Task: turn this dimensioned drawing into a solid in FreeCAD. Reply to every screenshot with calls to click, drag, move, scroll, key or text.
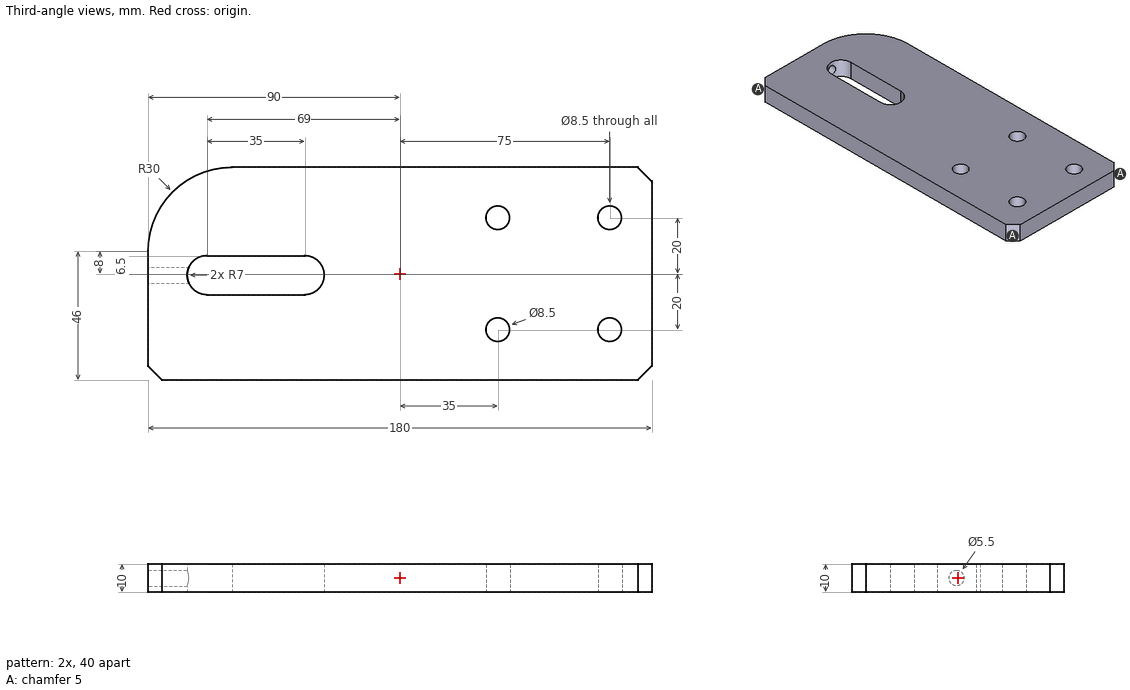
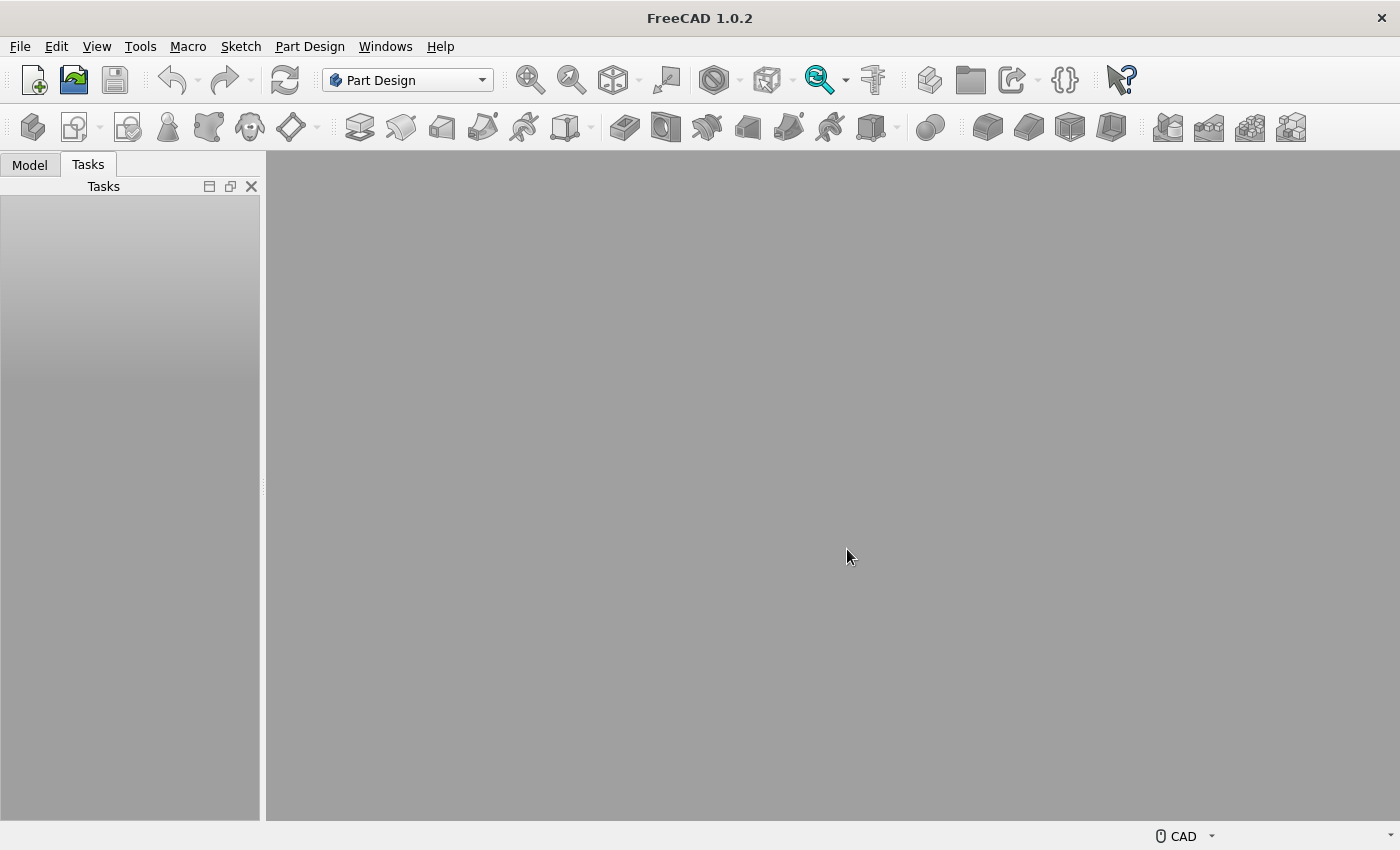
click(33, 80)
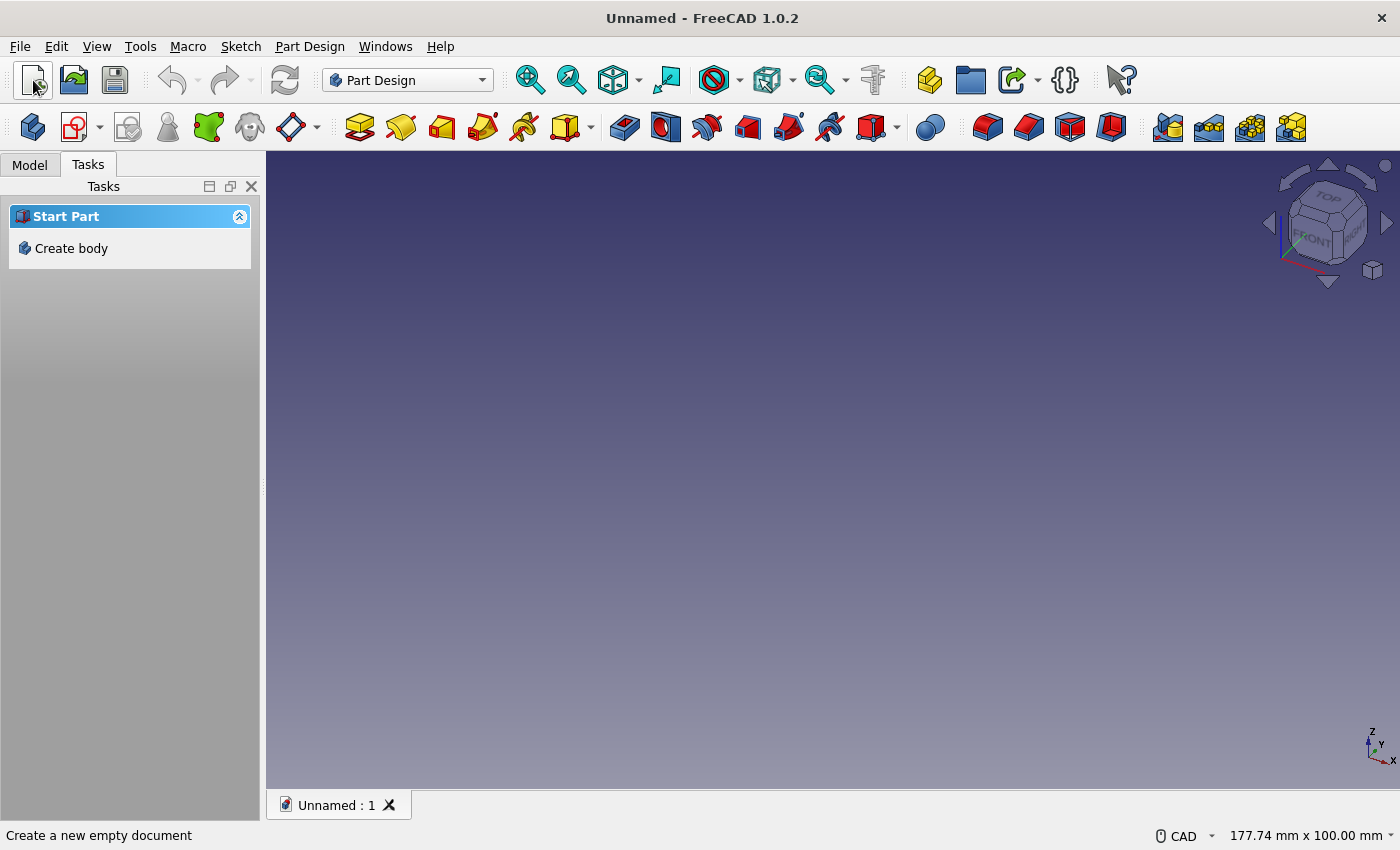
click(74, 128)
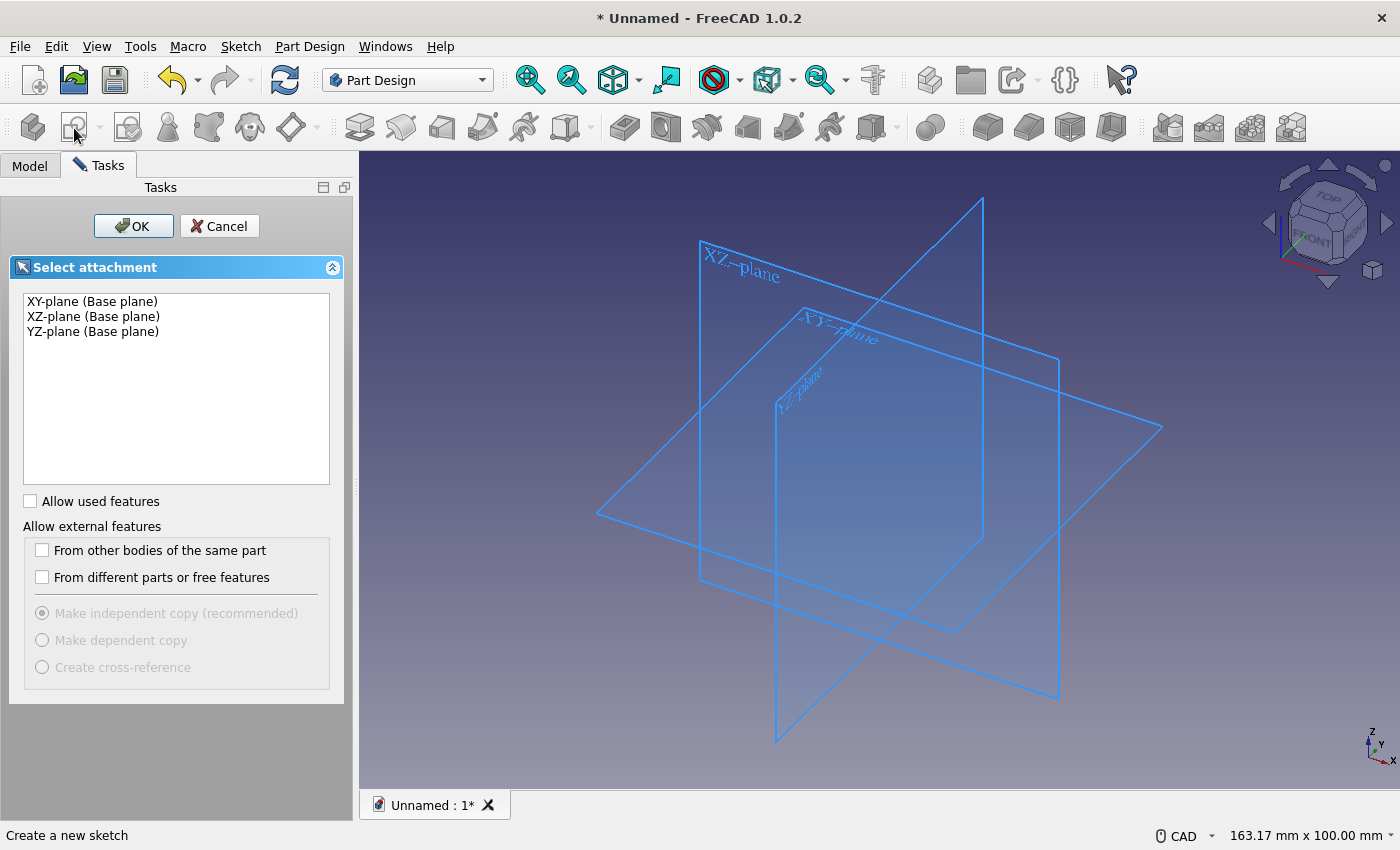
click(84, 302)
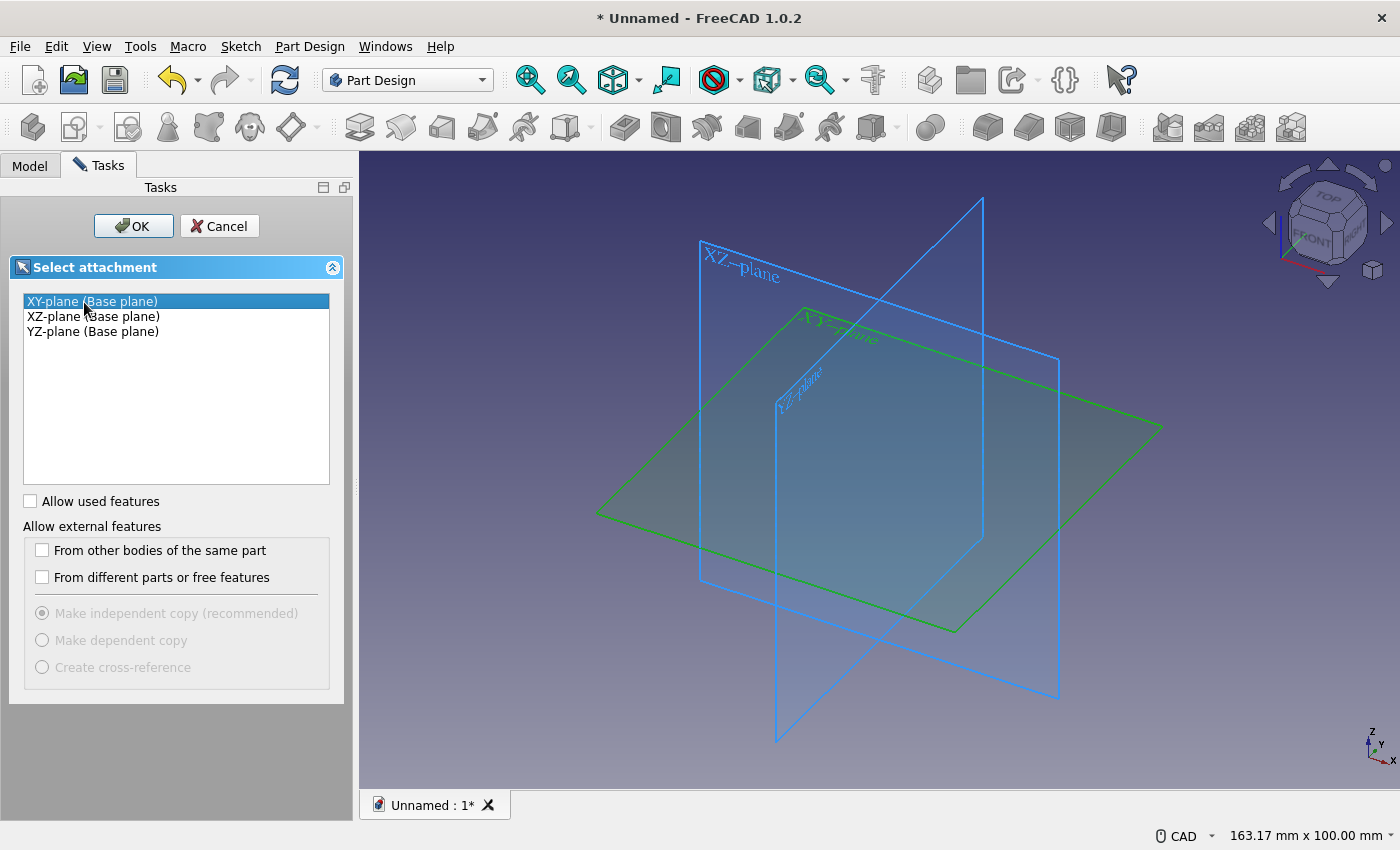
click(134, 226)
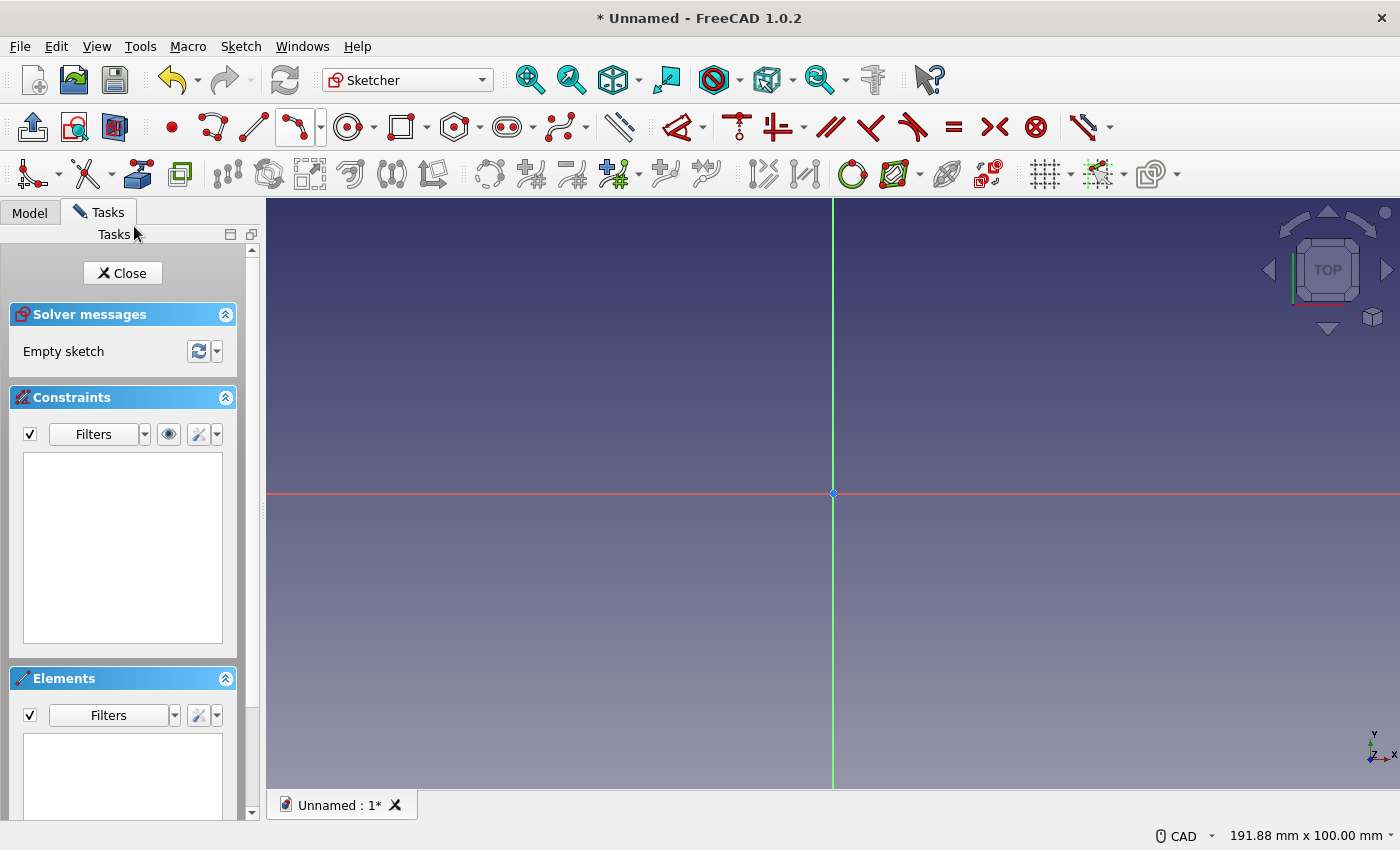
scroll(625, 494, down, 2)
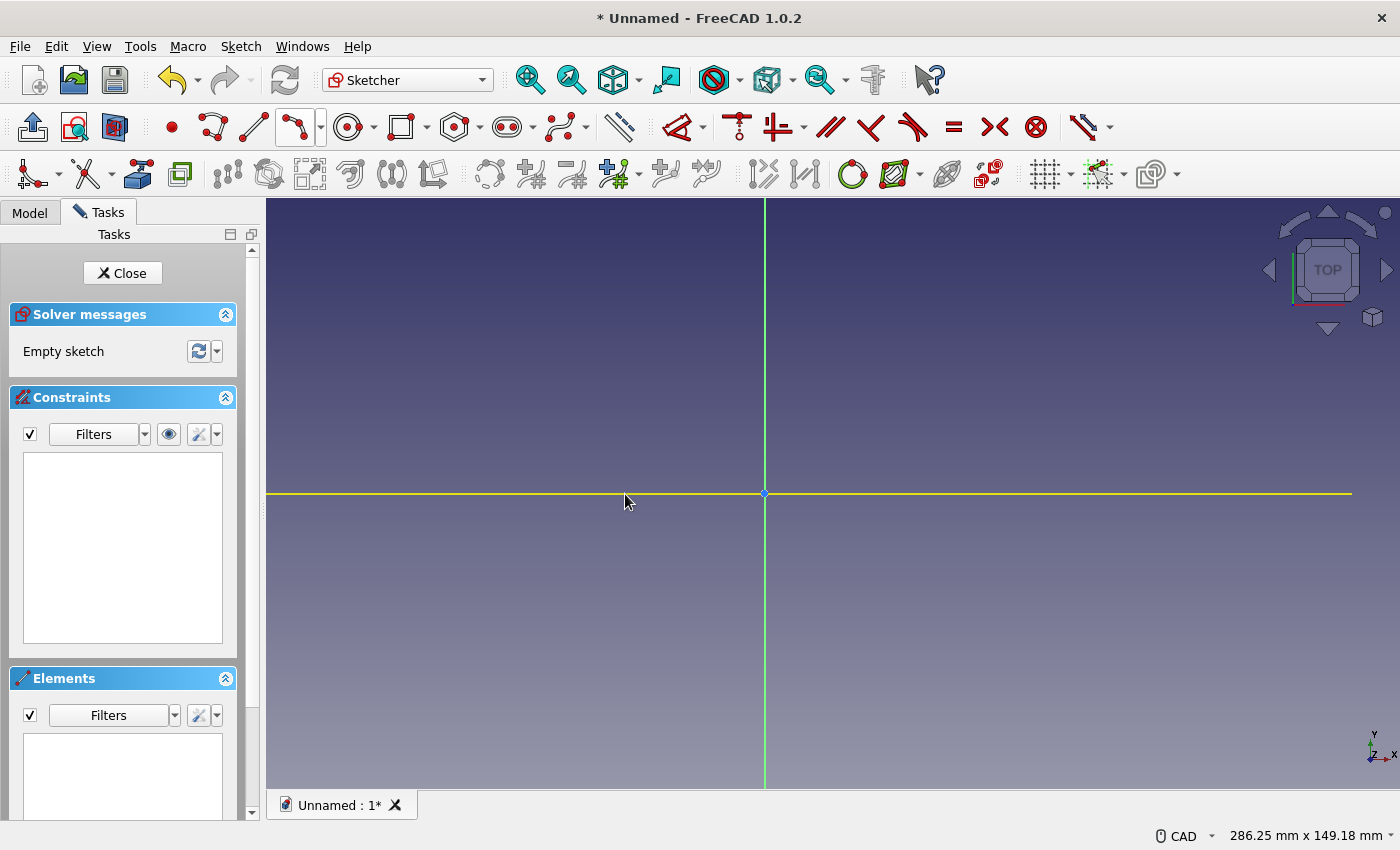
key(g)
key(m)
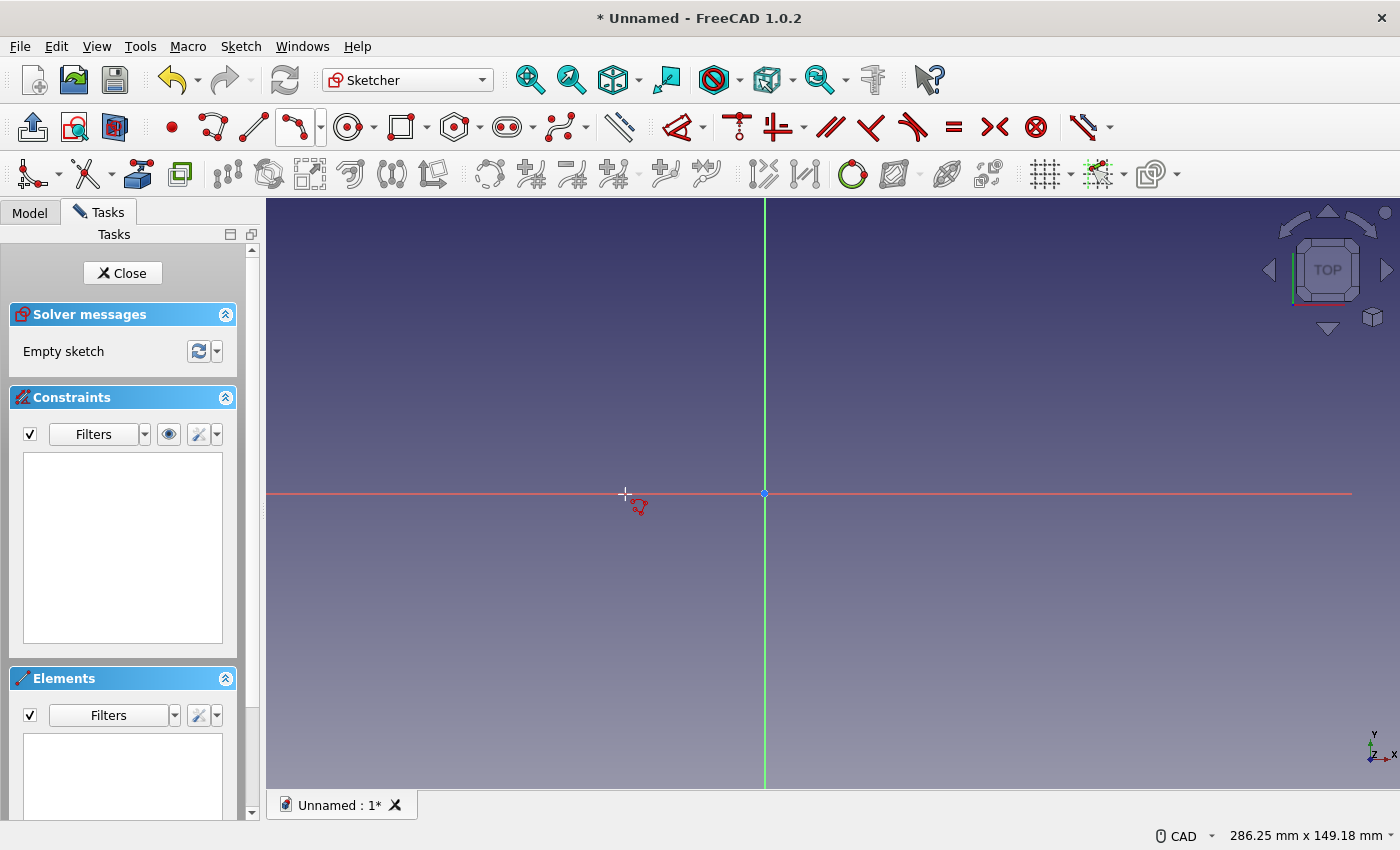
click(408, 462)
click(408, 644)
click(1121, 644)
click(1121, 343)
click(527, 343)
right_click(527, 343)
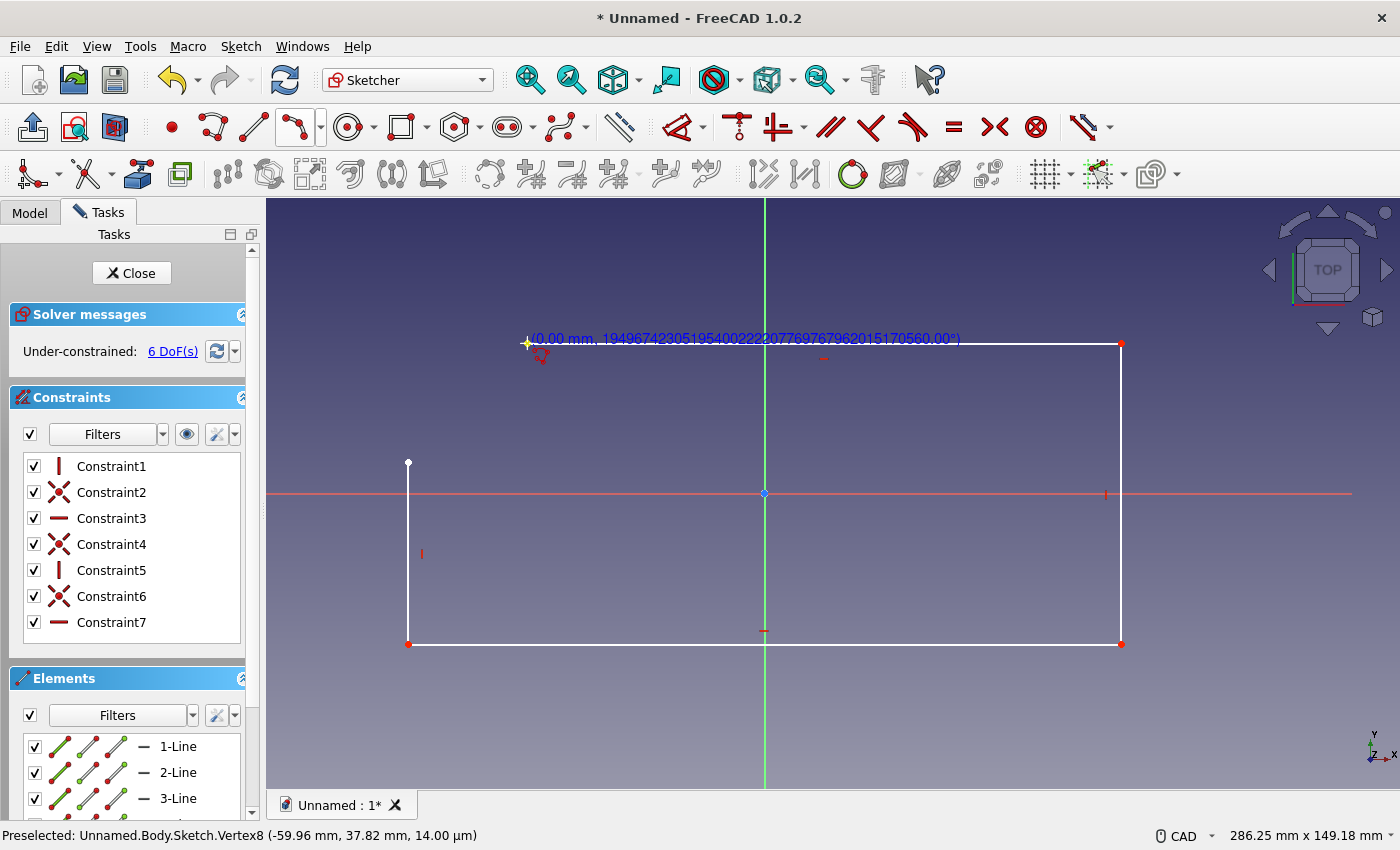
click(294, 128)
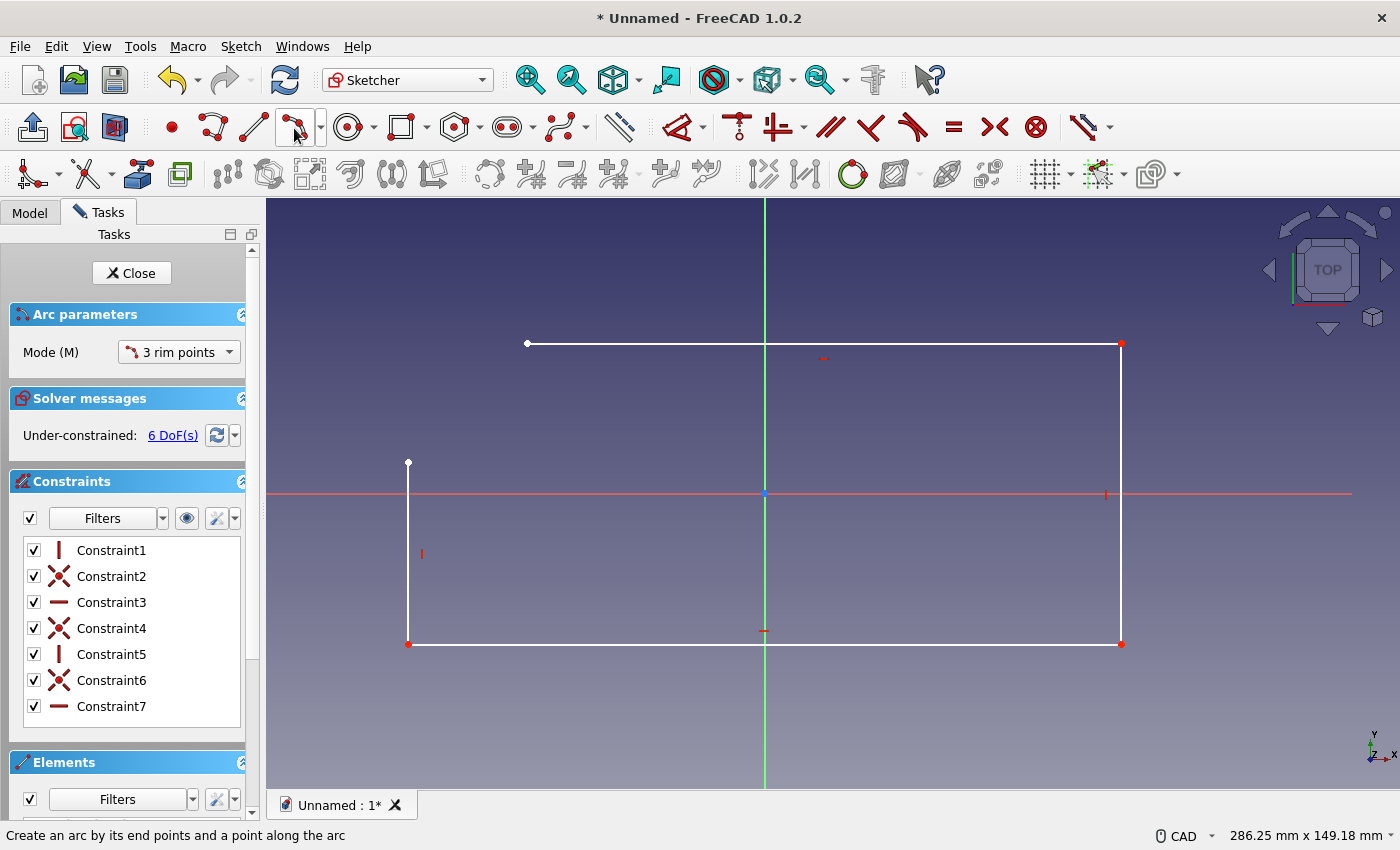
click(527, 344)
click(408, 463)
click(443, 378)
key(Escape)